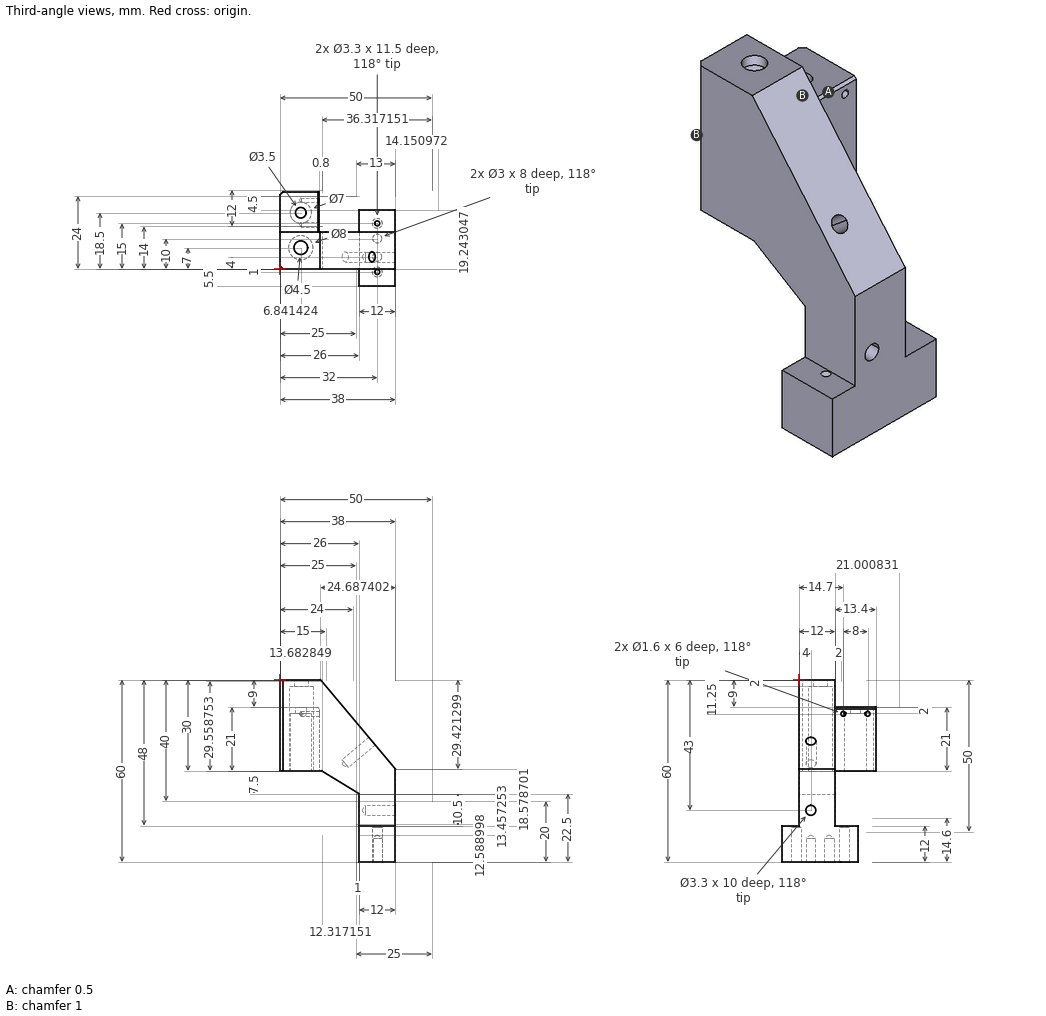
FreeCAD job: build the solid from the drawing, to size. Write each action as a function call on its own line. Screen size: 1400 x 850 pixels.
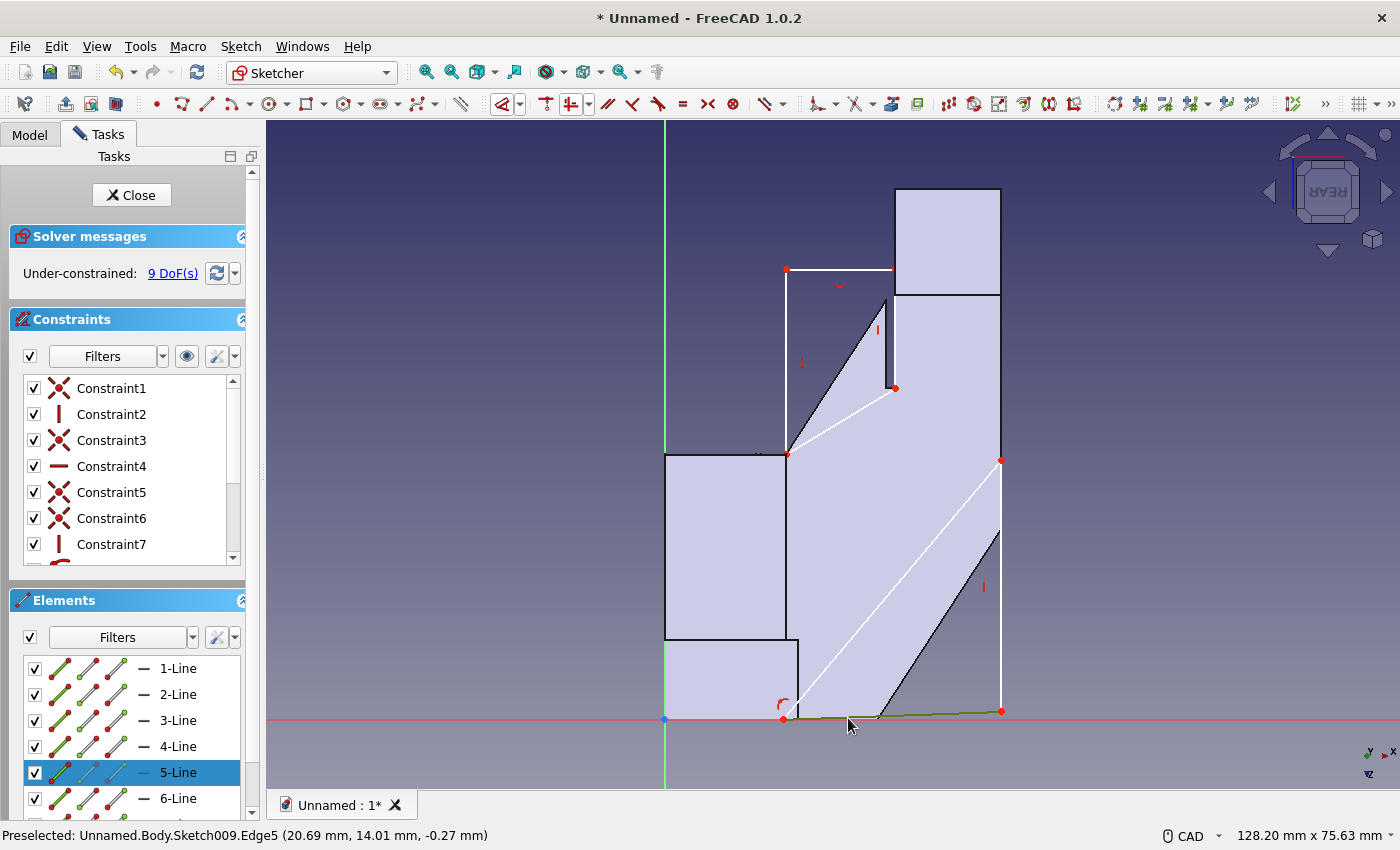
click(588, 104)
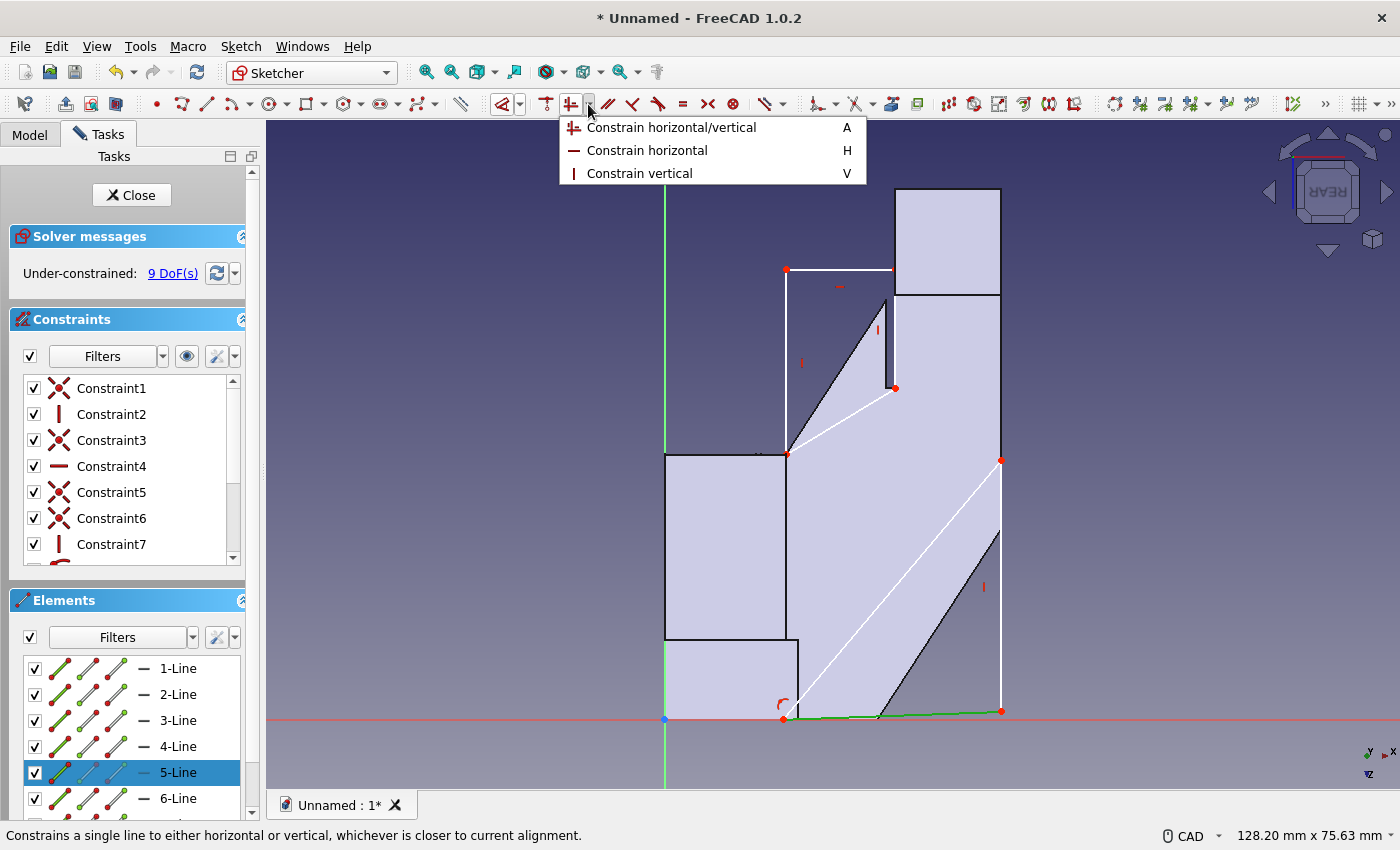
click(713, 150)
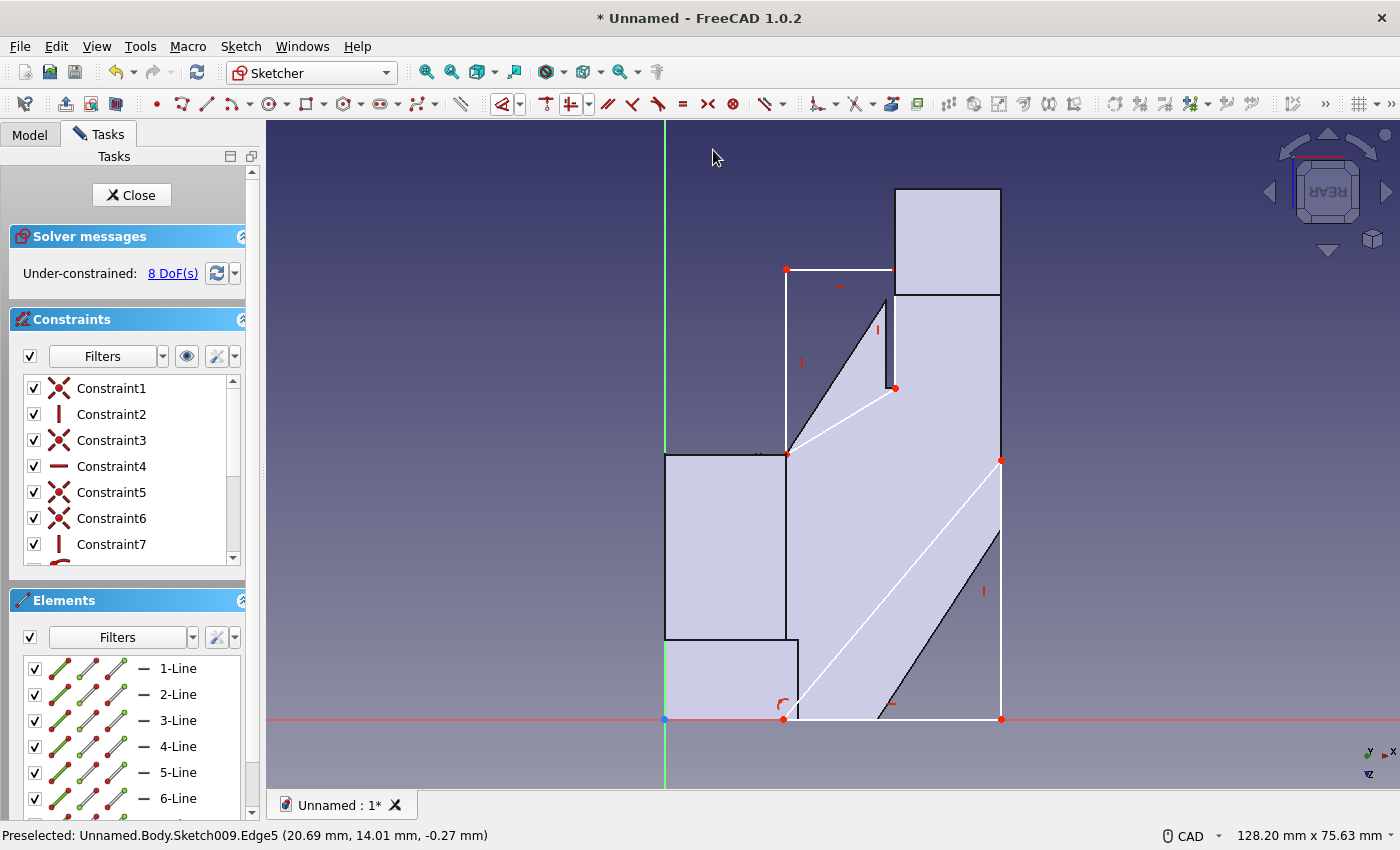
click(786, 455)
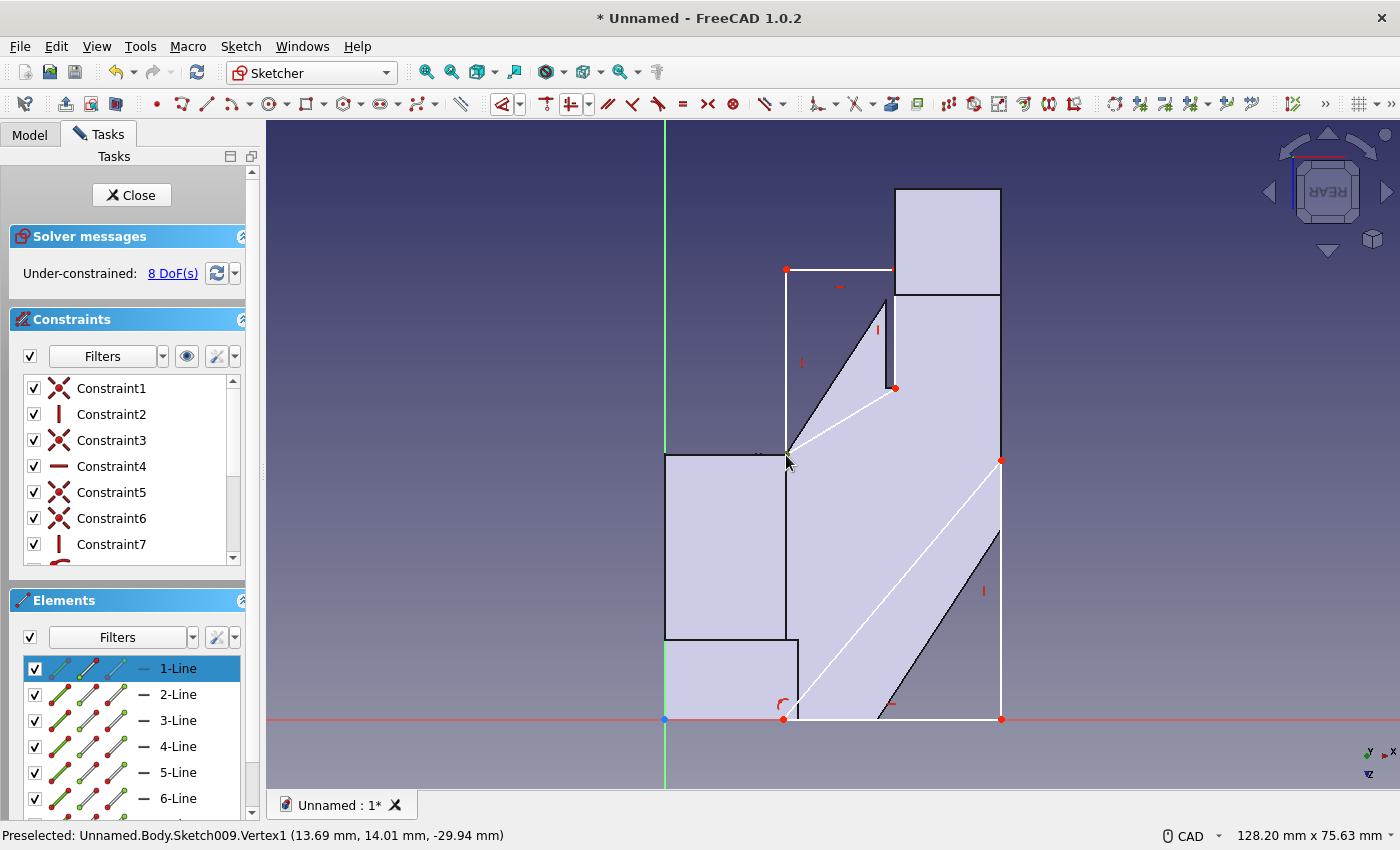
key(i)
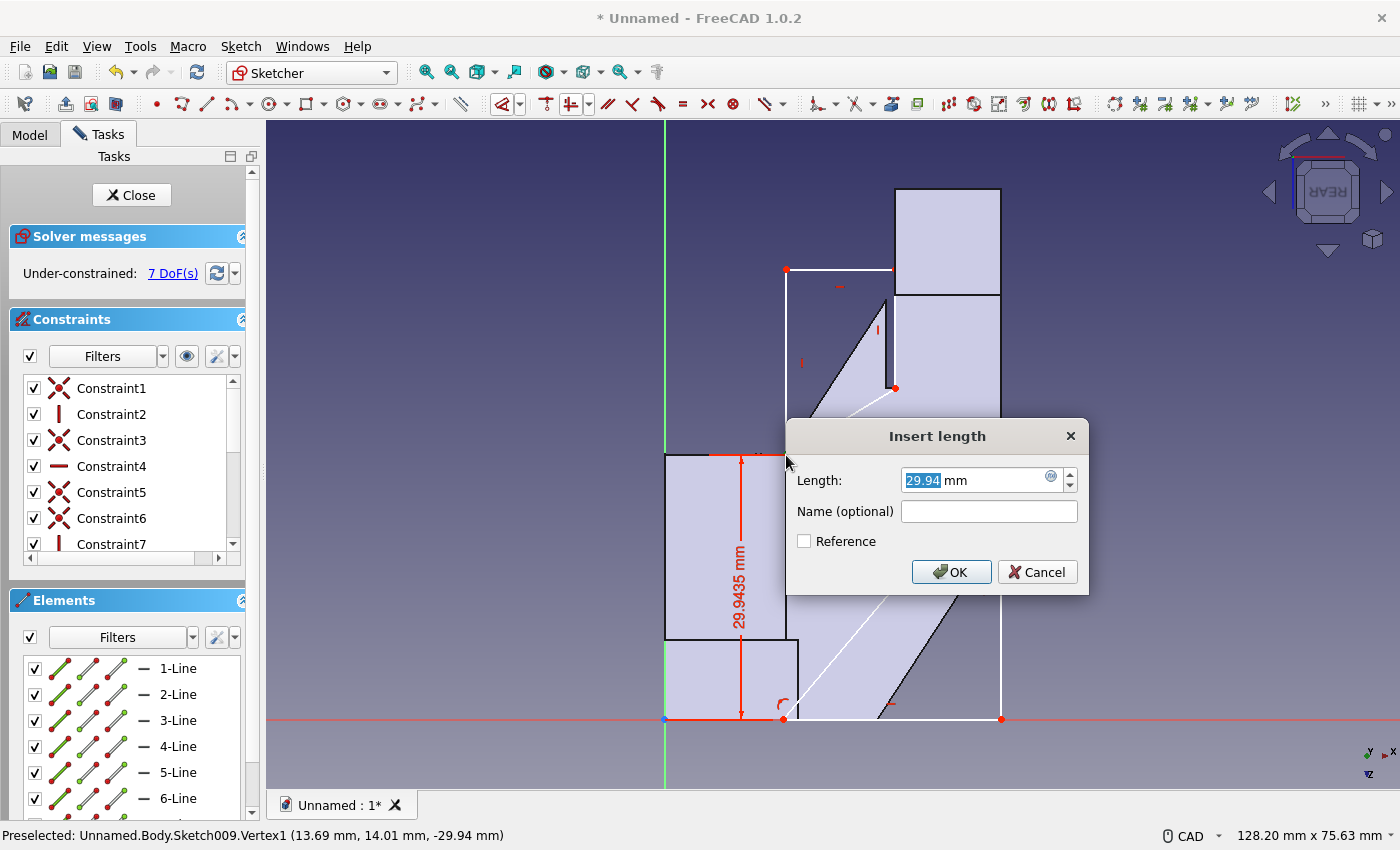
text(30)
key(Return)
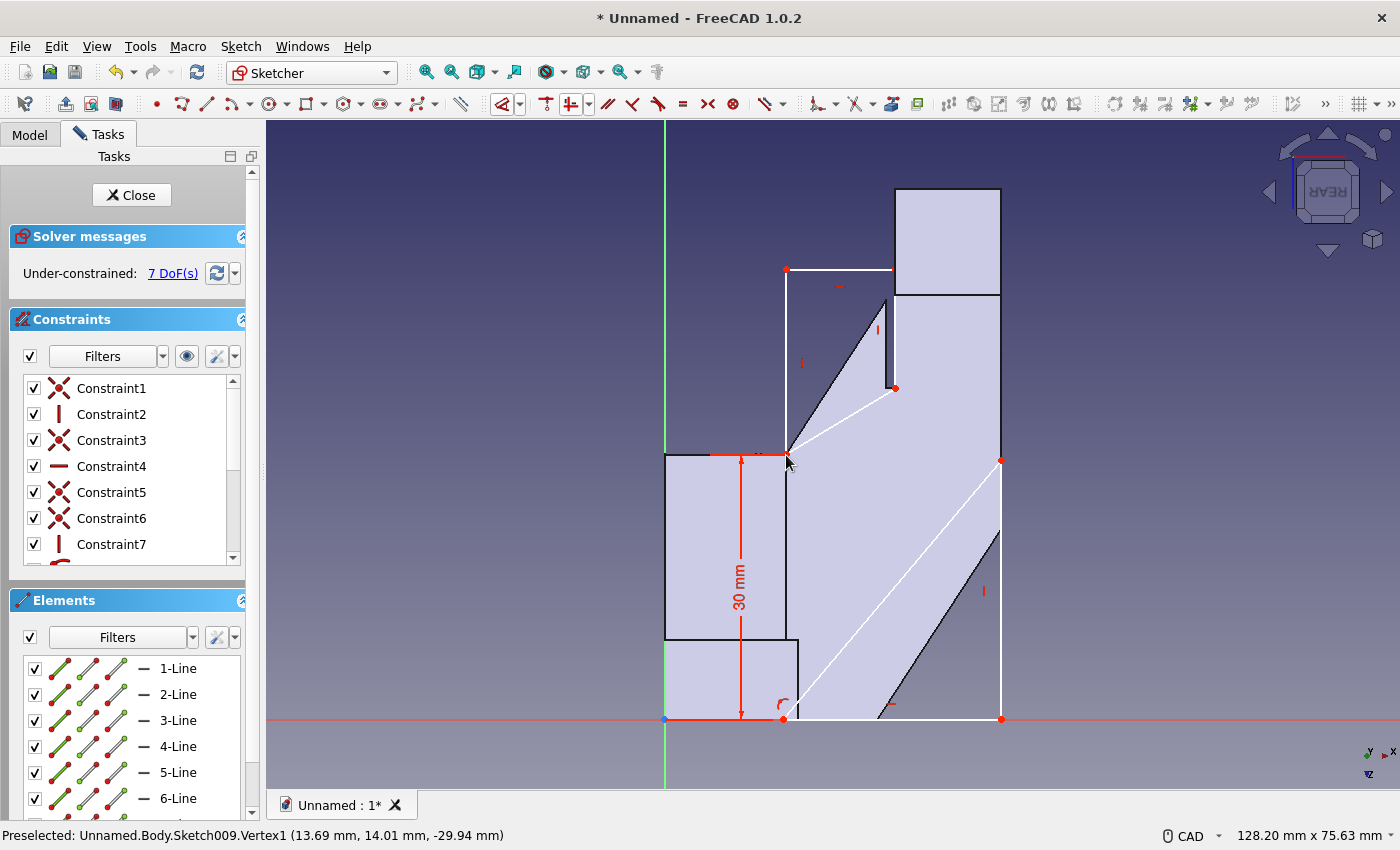
click(895, 389)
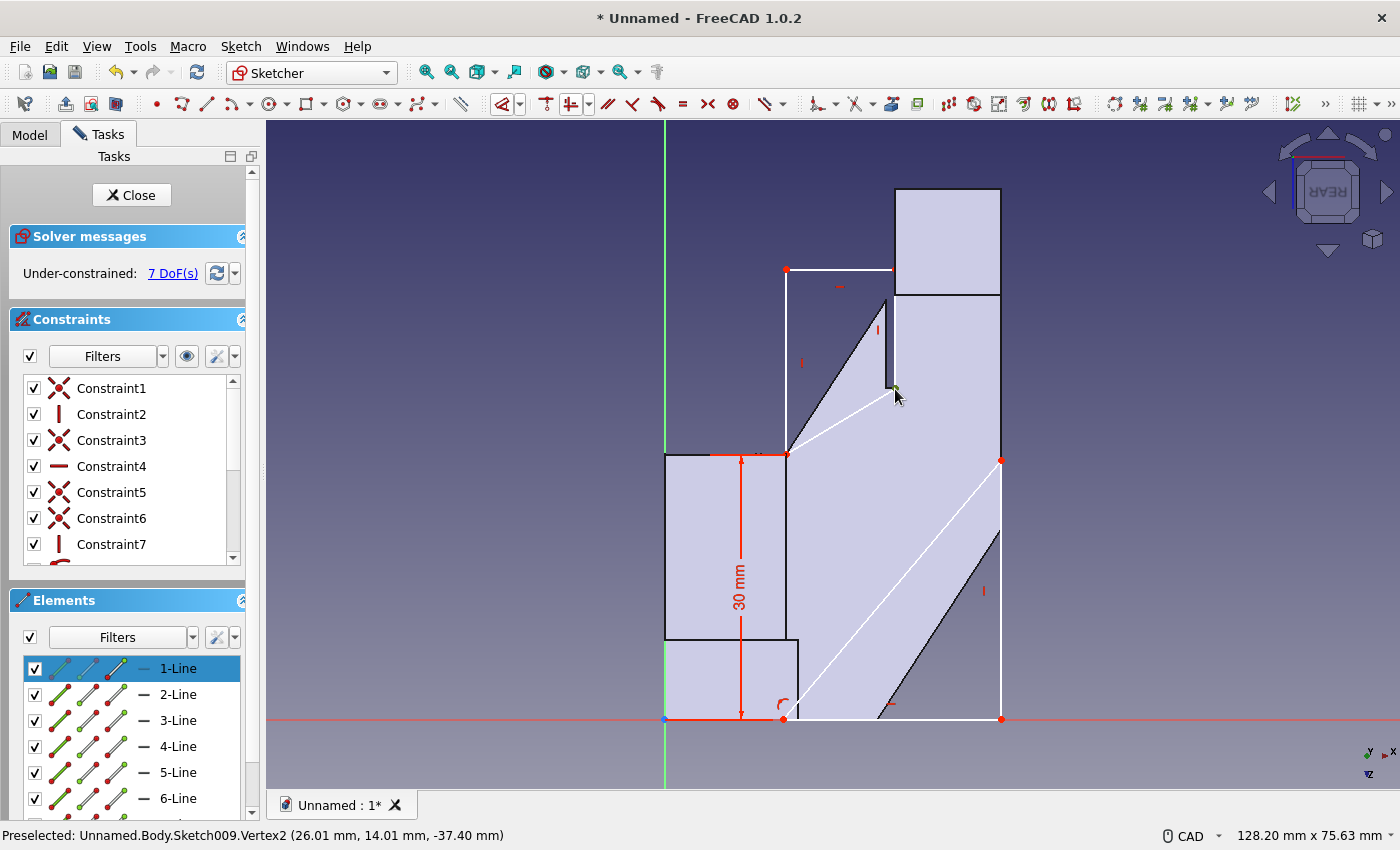
click(520, 104)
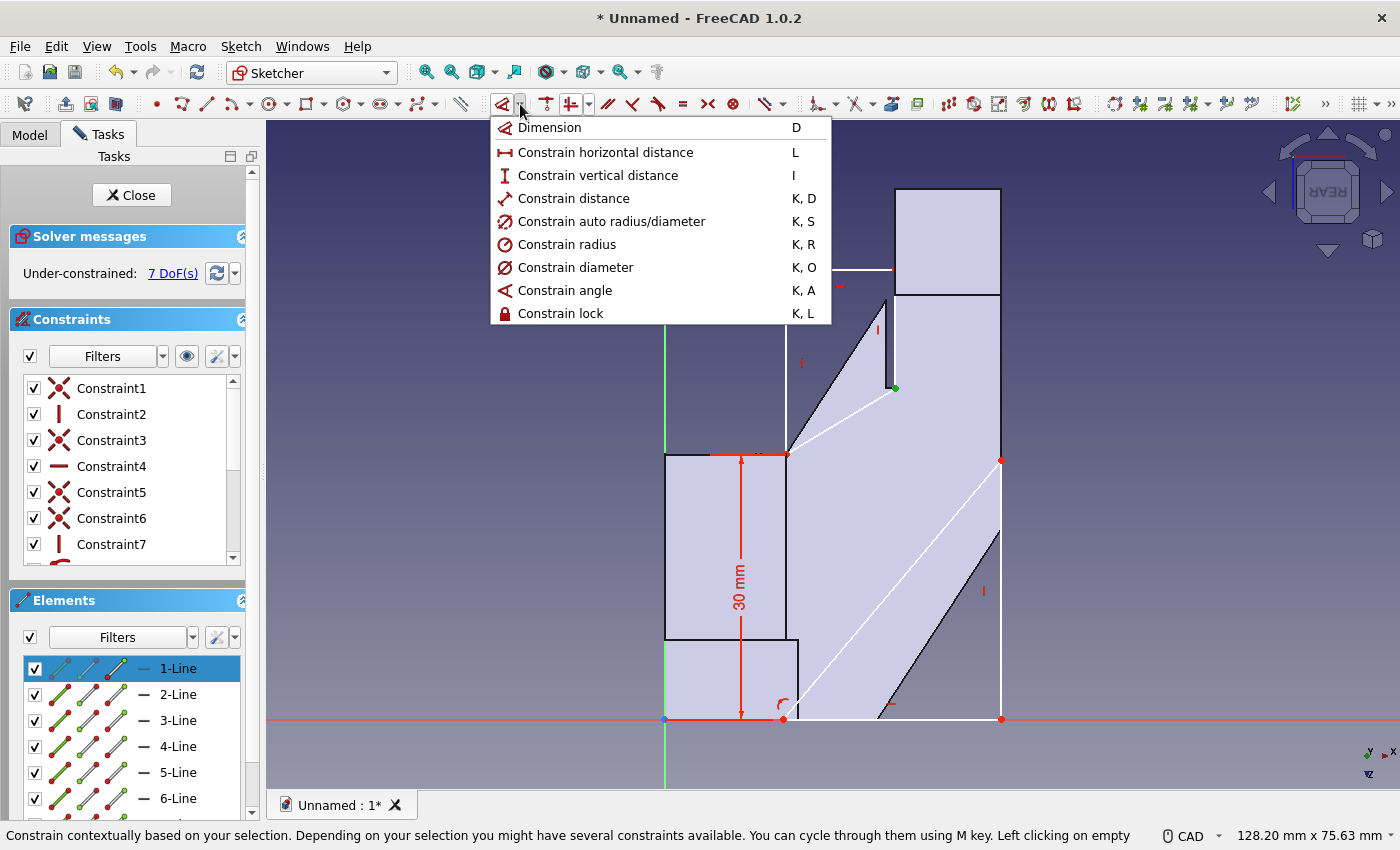
click(661, 152)